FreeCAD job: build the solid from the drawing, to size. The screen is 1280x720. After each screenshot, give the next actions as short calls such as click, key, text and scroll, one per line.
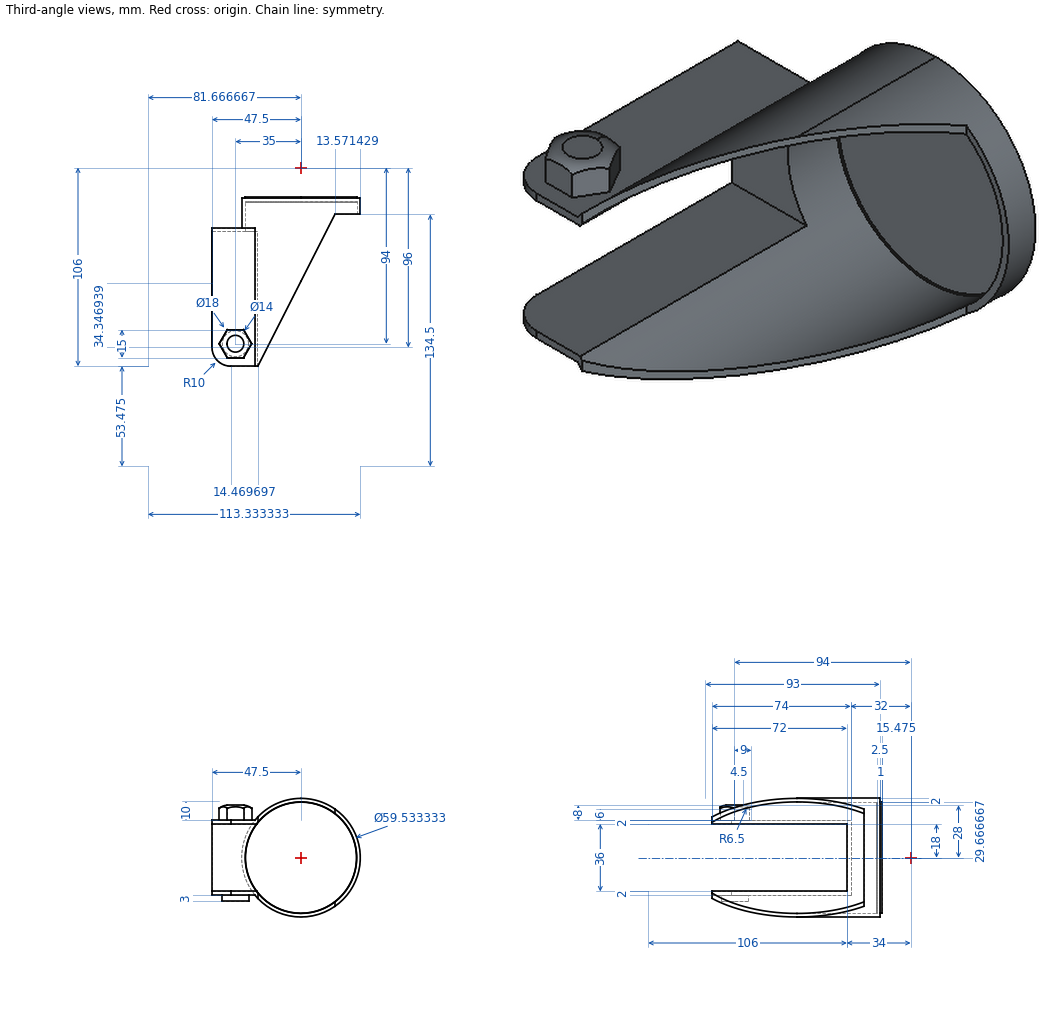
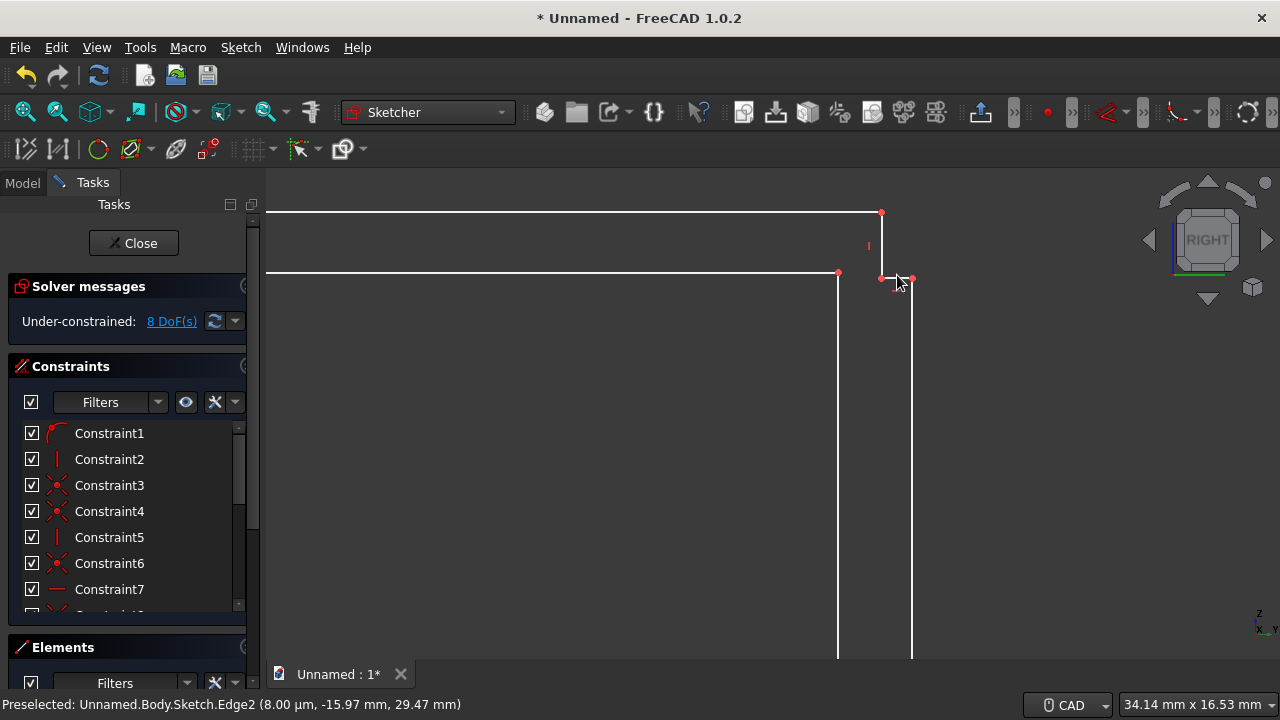
scroll(894, 361, down, 9)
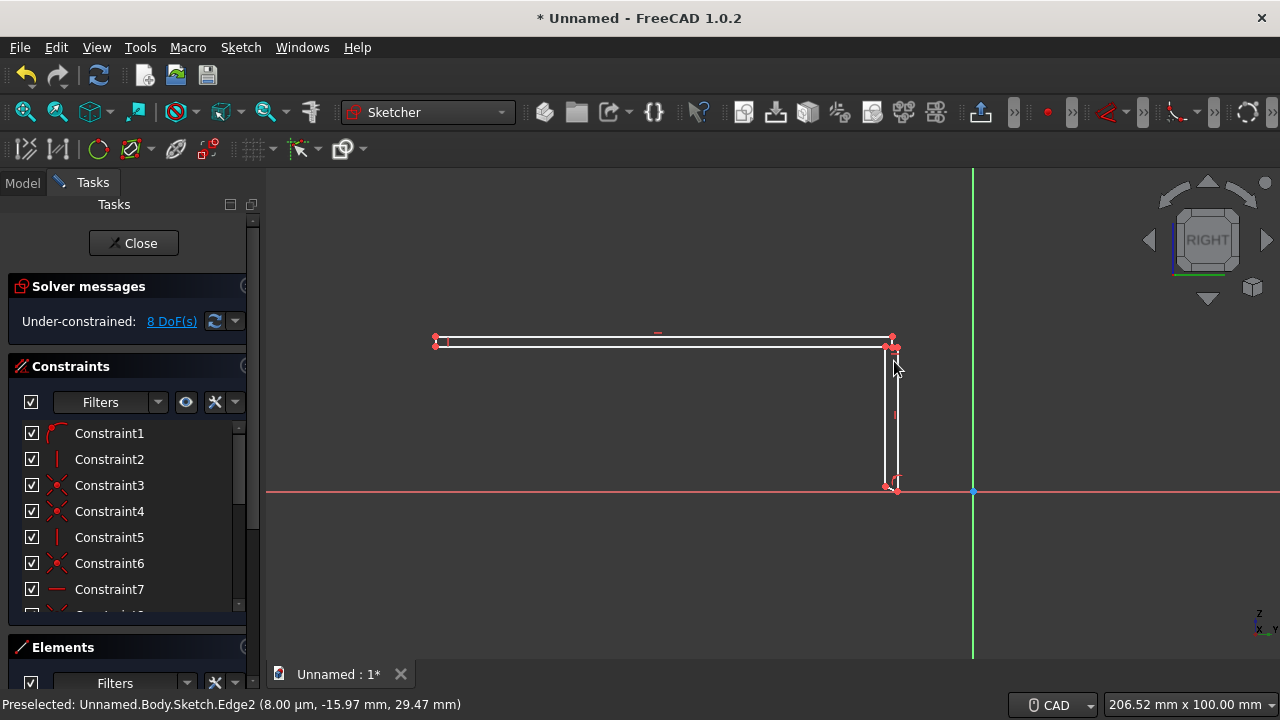
scroll(889, 488, up, 7)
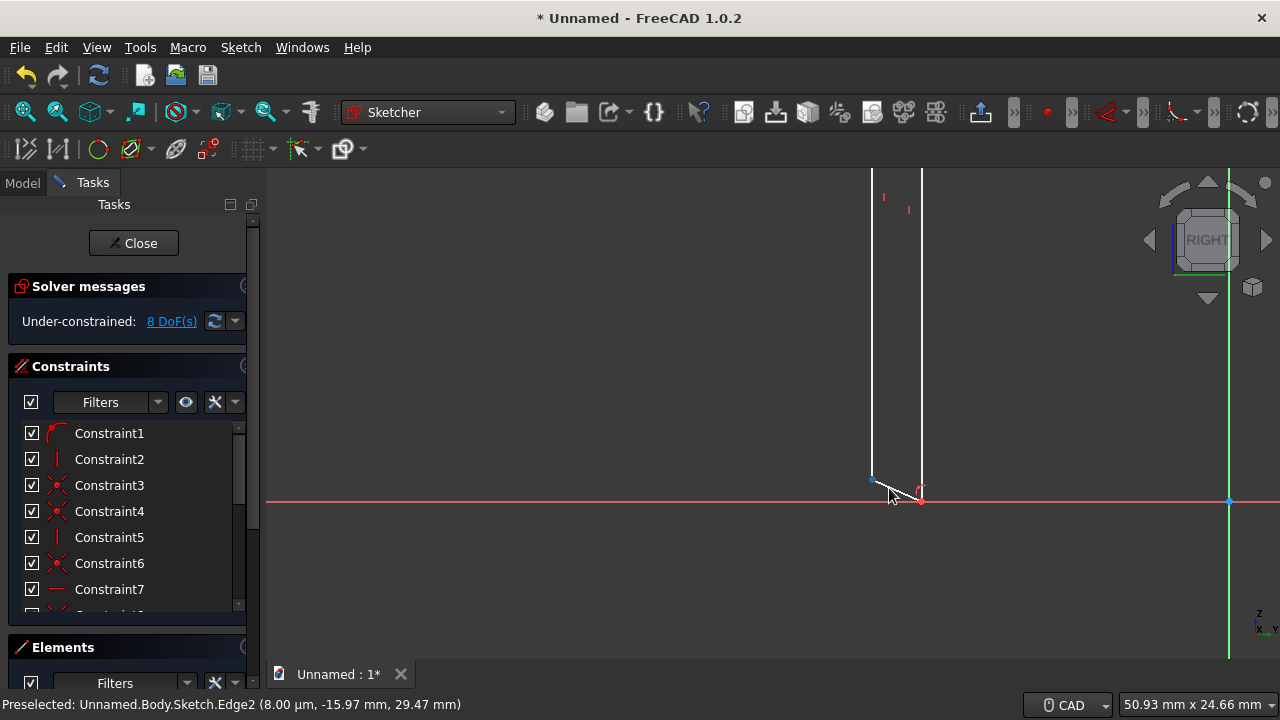
click(887, 486)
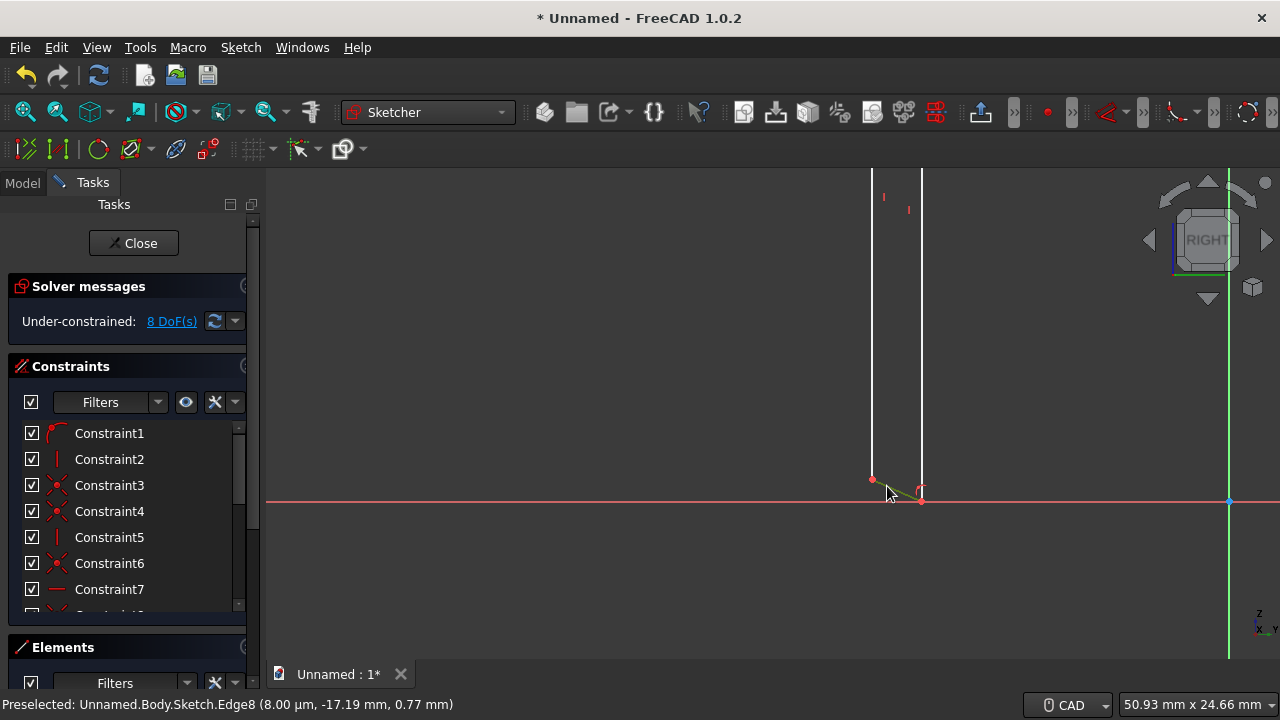
key(h)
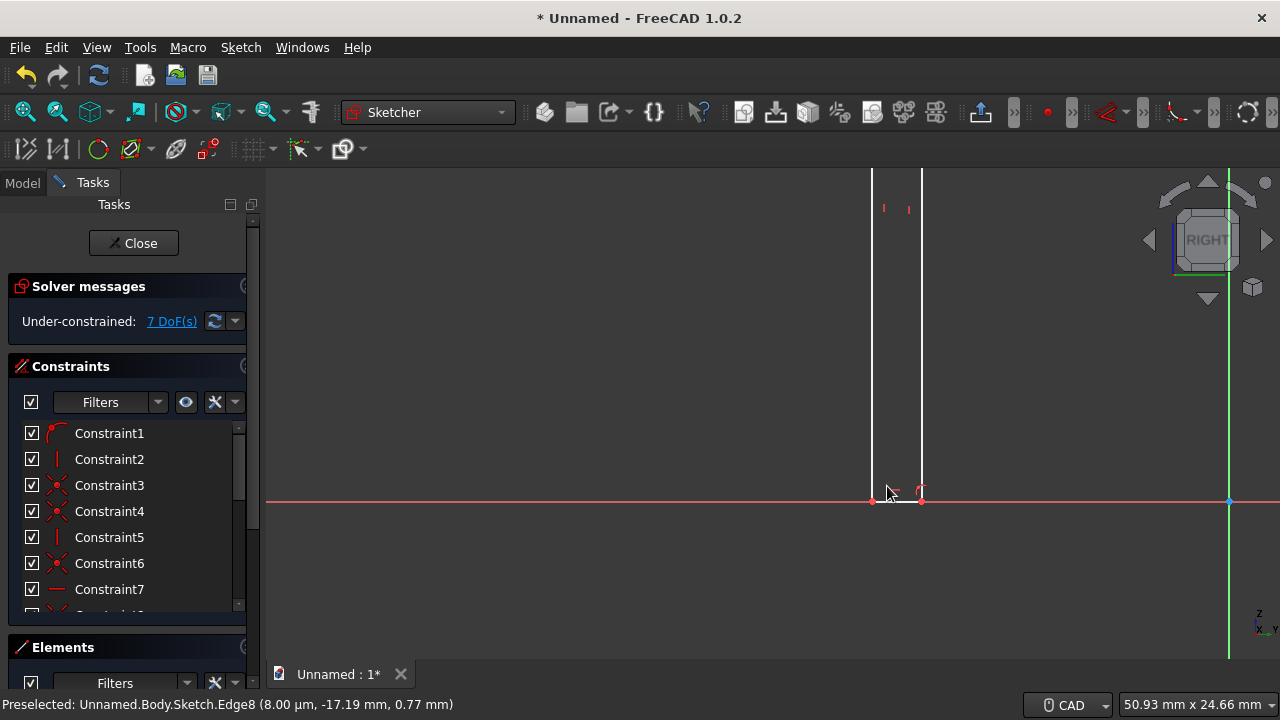
click(1106, 112)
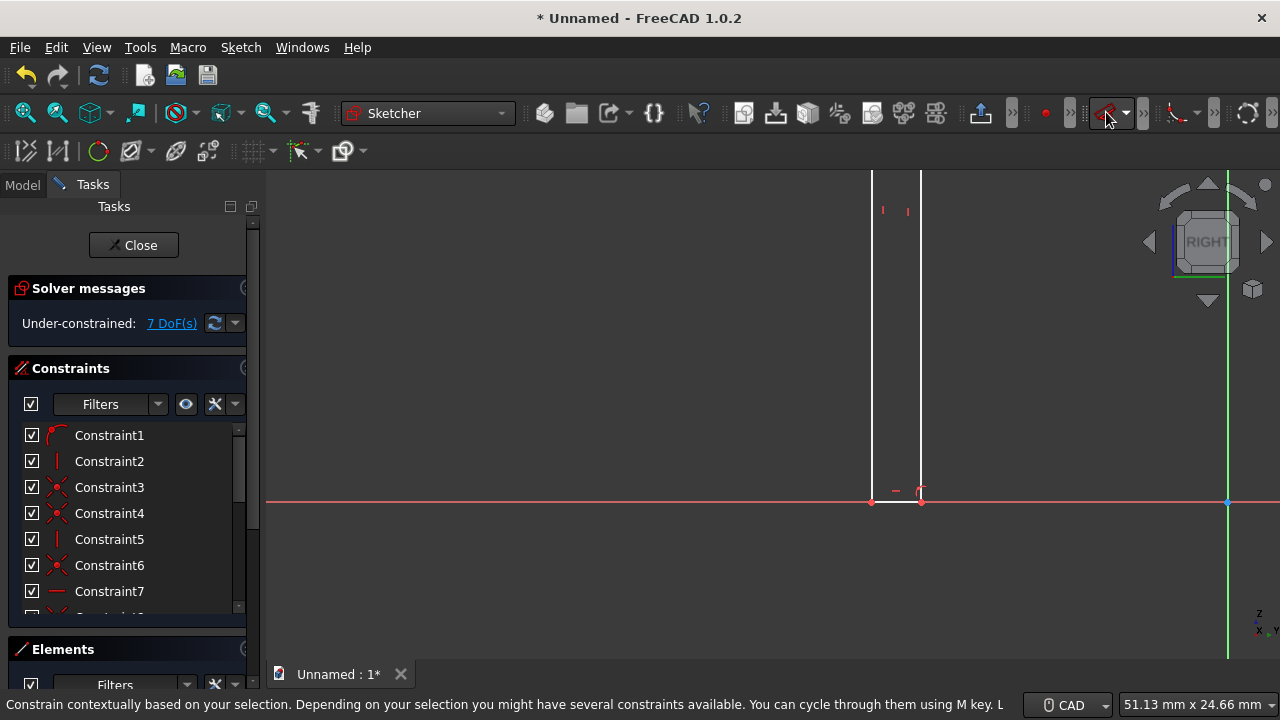
scroll(889, 489, down, 7)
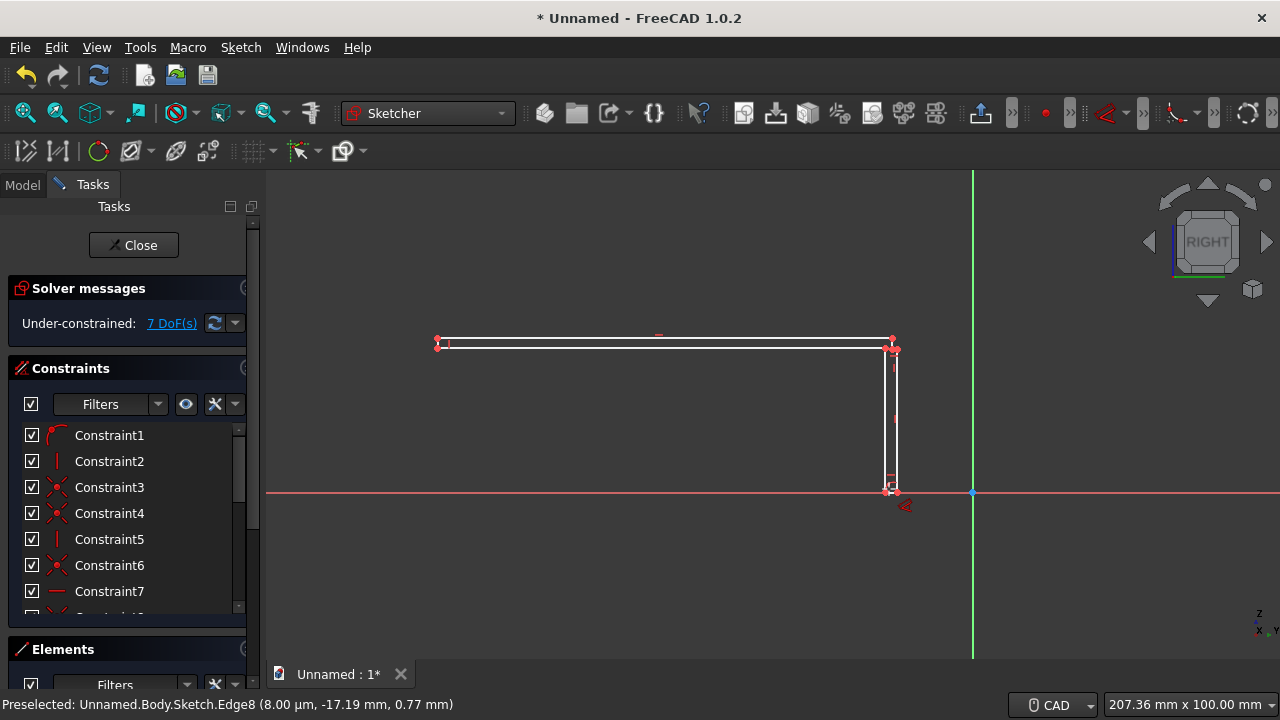
scroll(895, 349, up, 11)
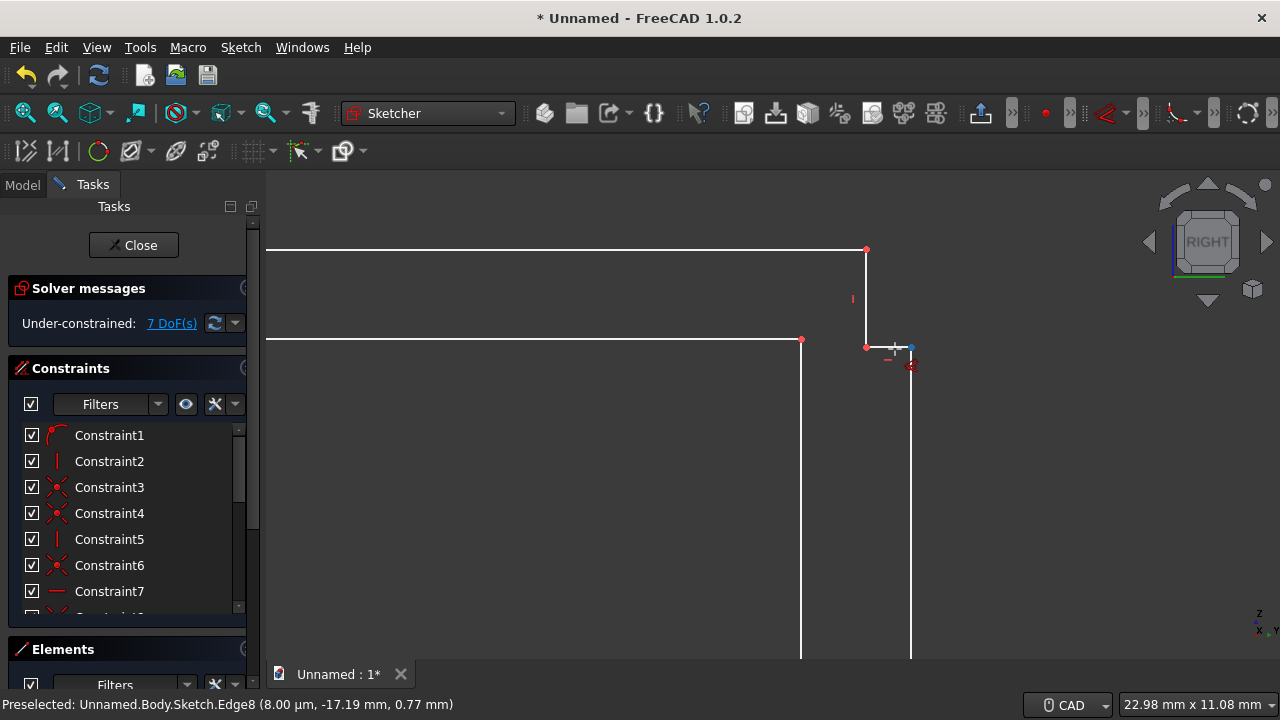
click(889, 347)
click(889, 313)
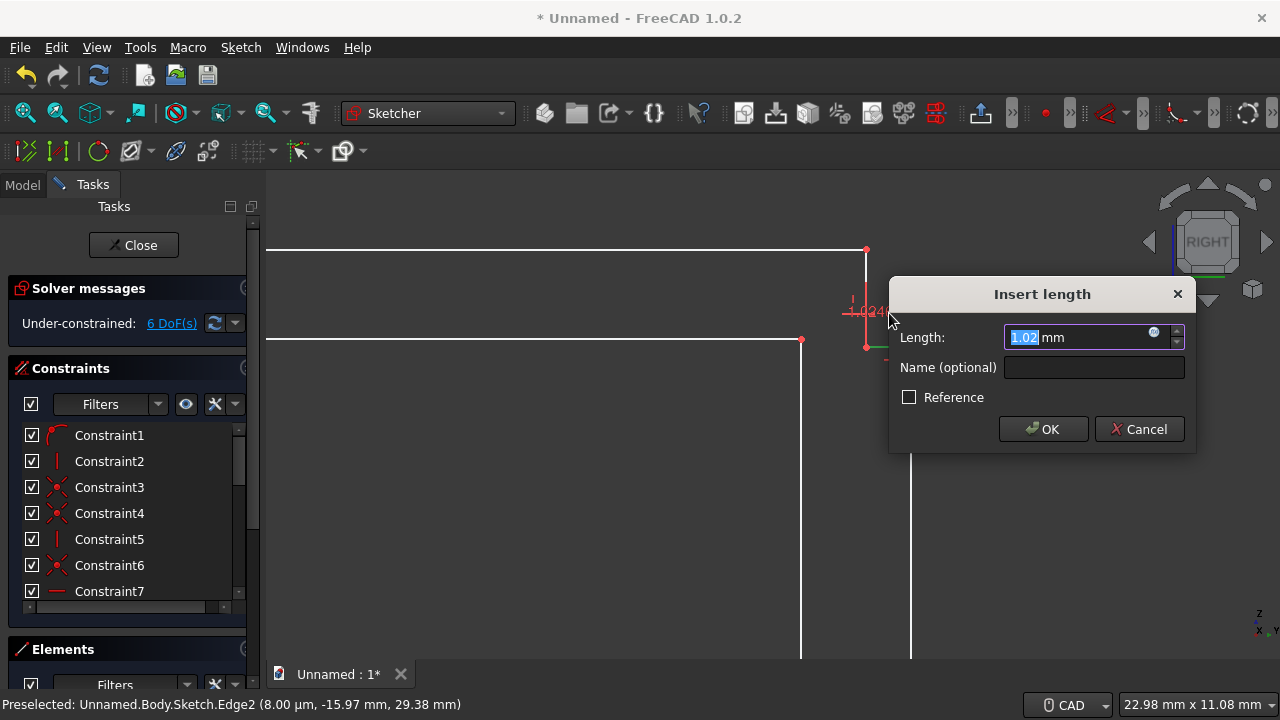
text(1)
key(Return)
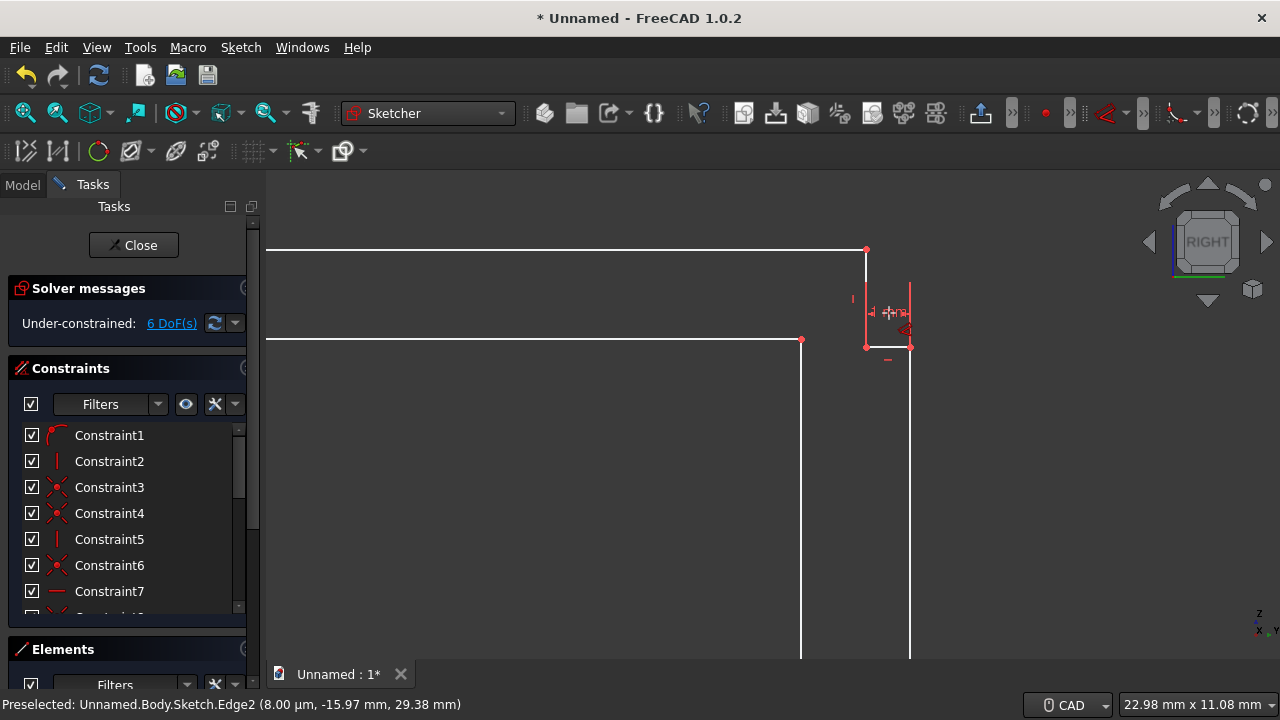
click(866, 318)
click(900, 276)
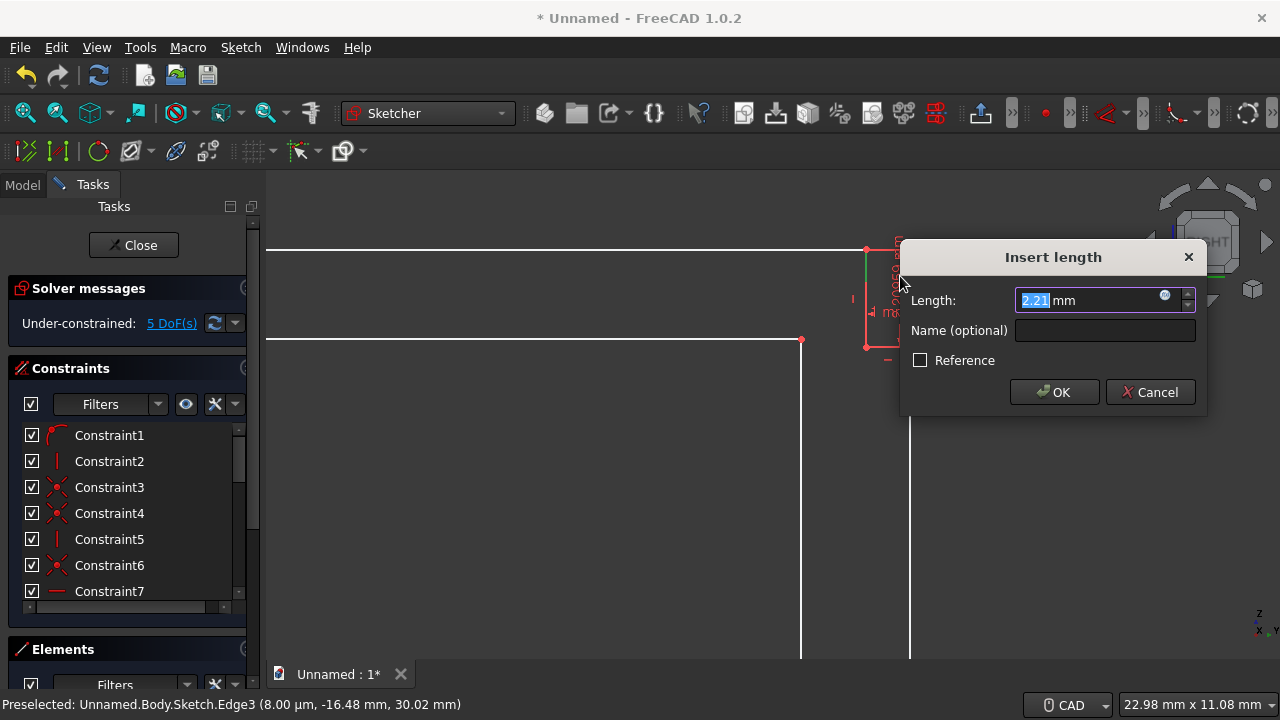
text(2)
key(Return)